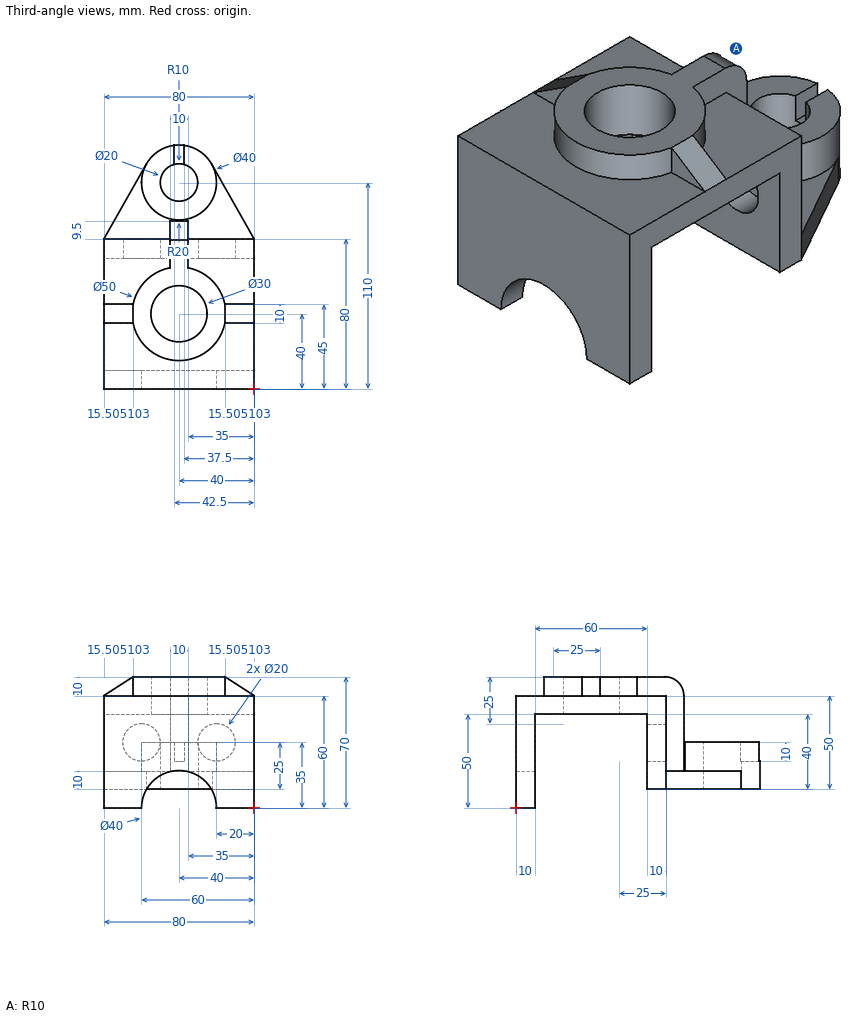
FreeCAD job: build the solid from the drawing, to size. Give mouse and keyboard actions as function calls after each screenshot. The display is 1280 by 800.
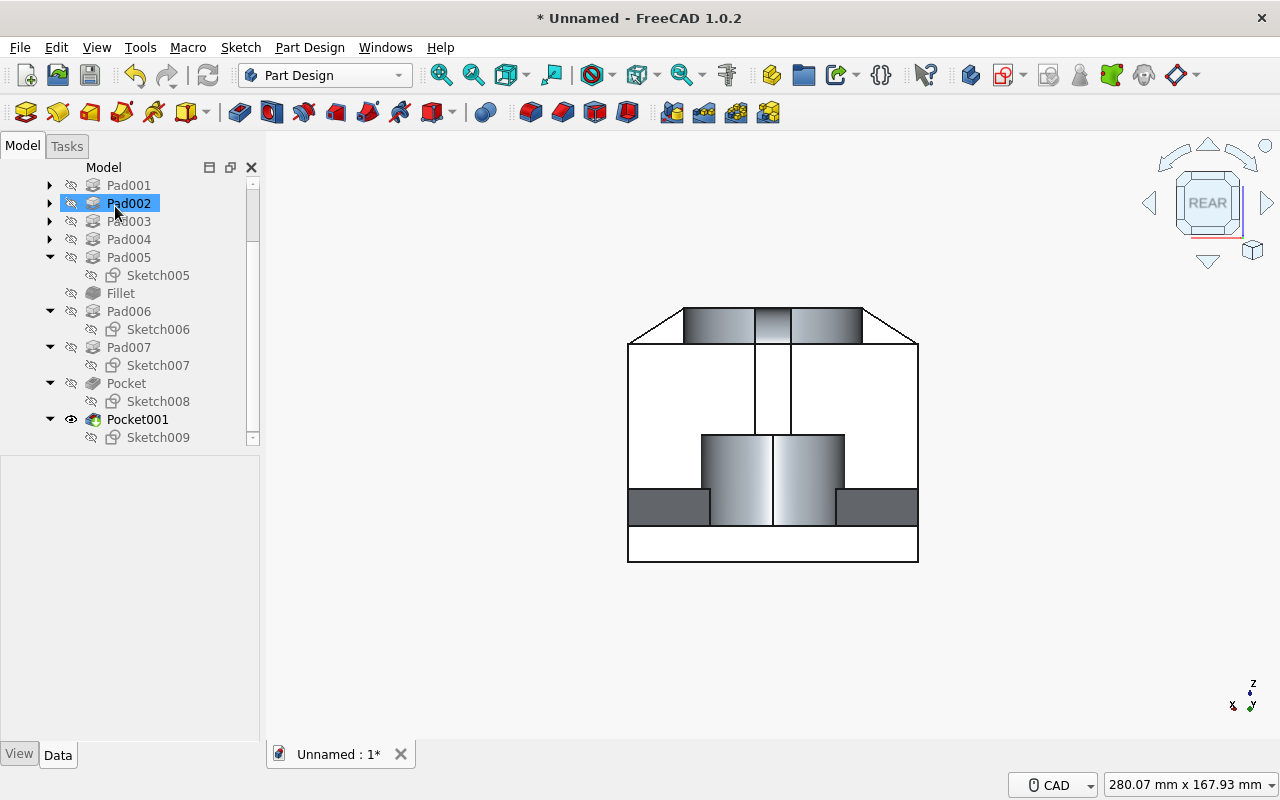
click(442, 76)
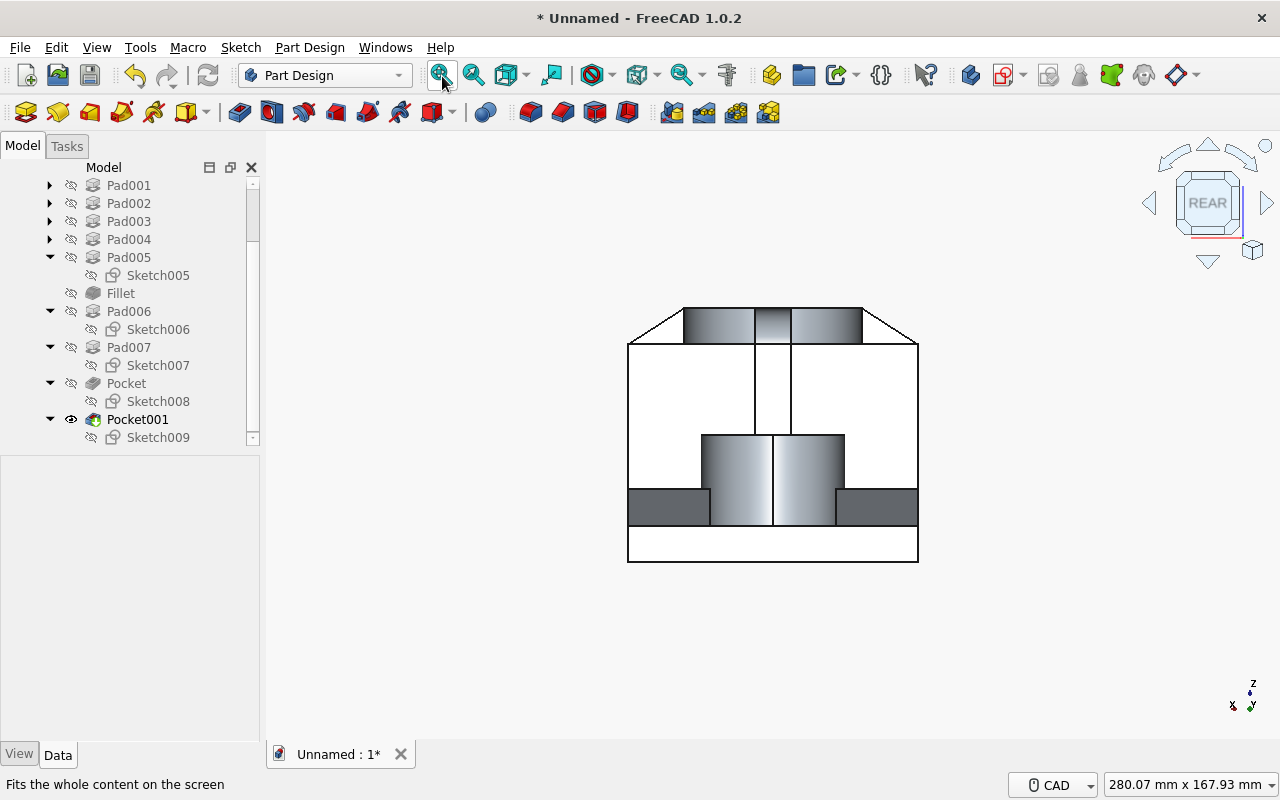
click(692, 416)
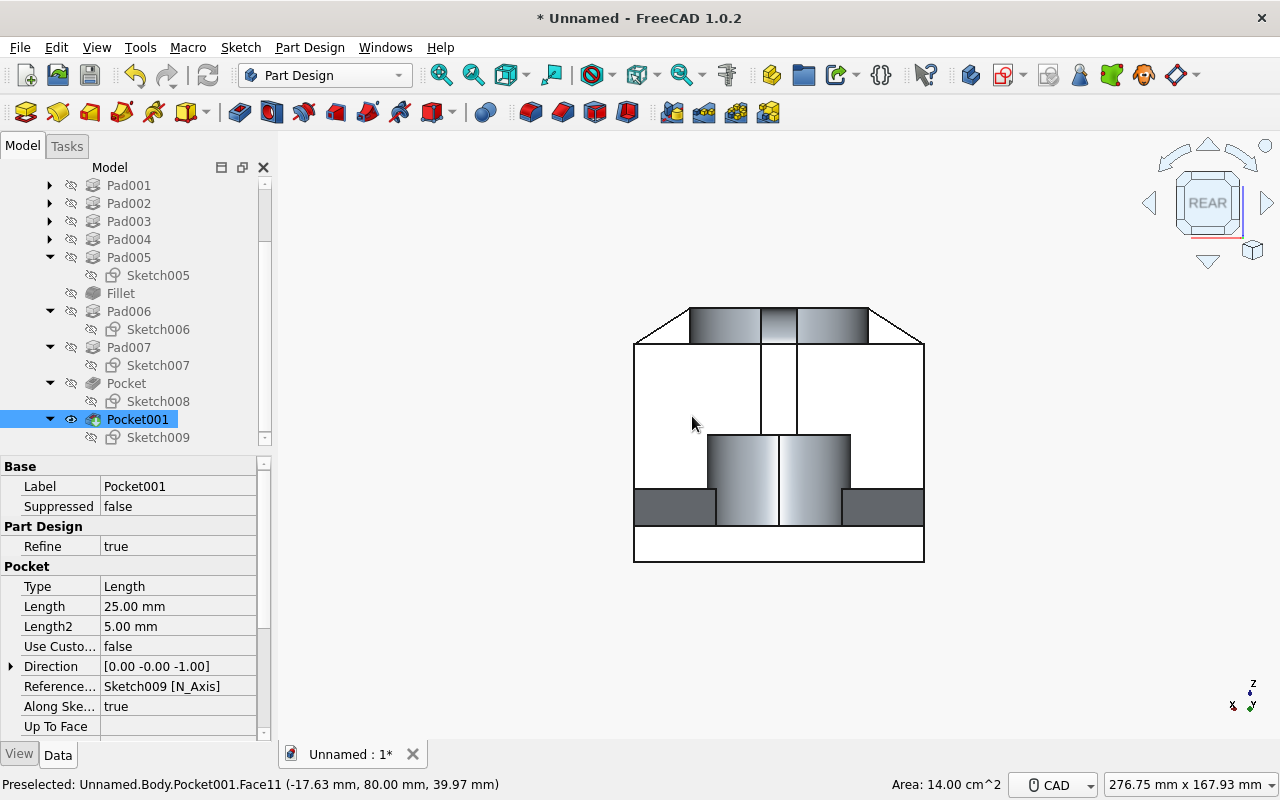
click(1004, 76)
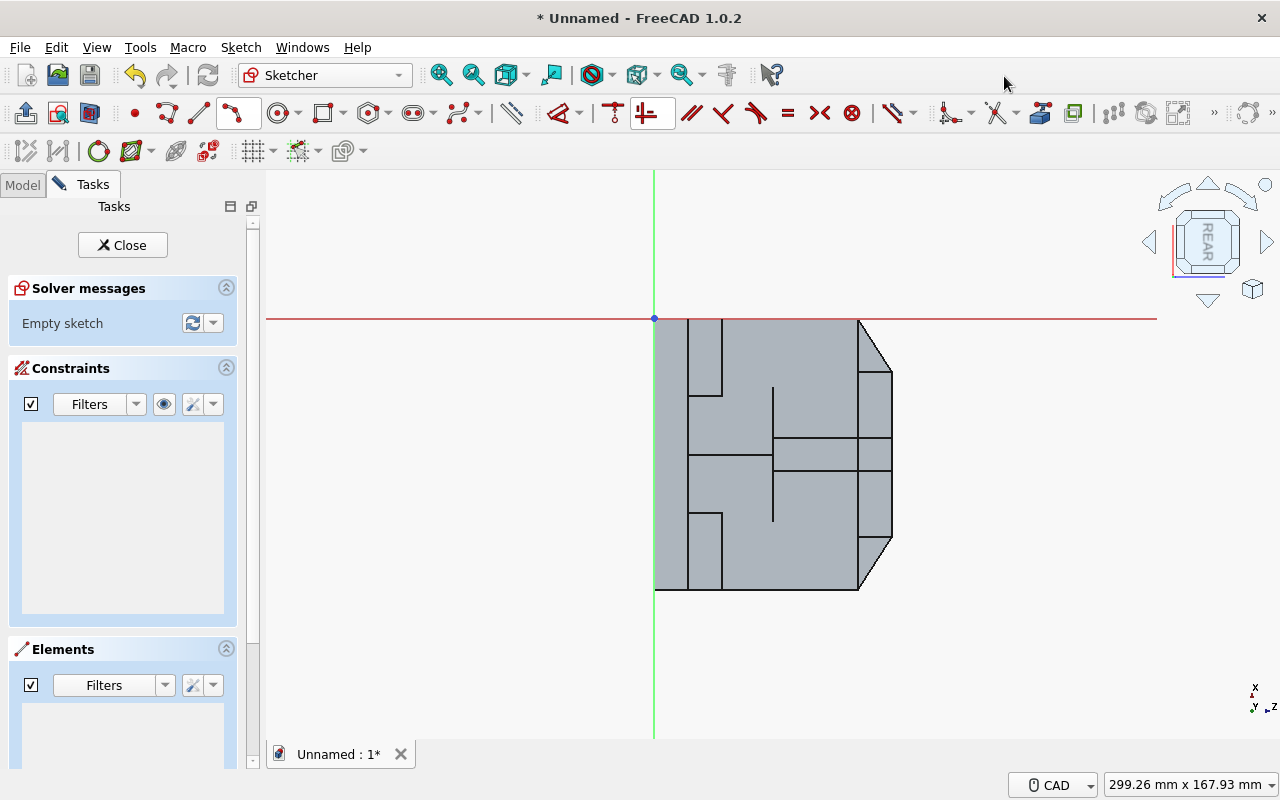
scroll(784, 403, up, 2)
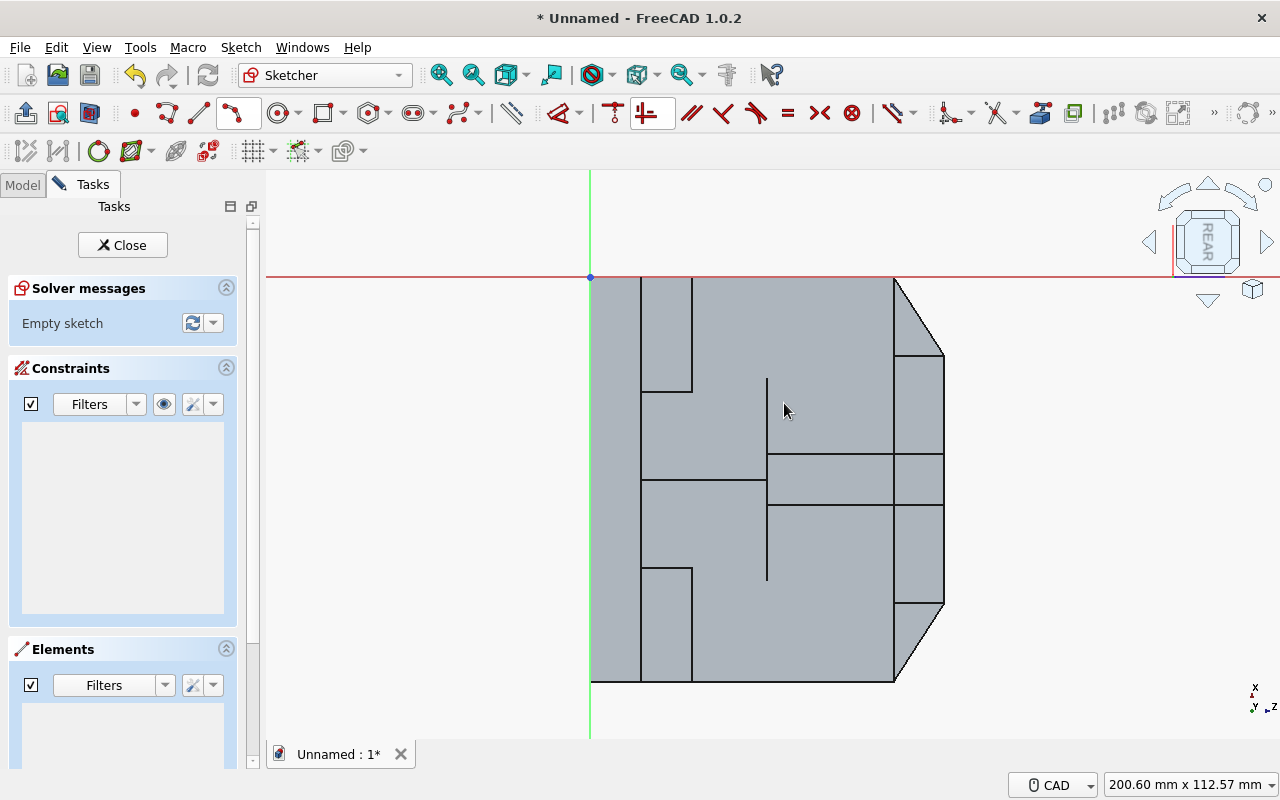
click(278, 114)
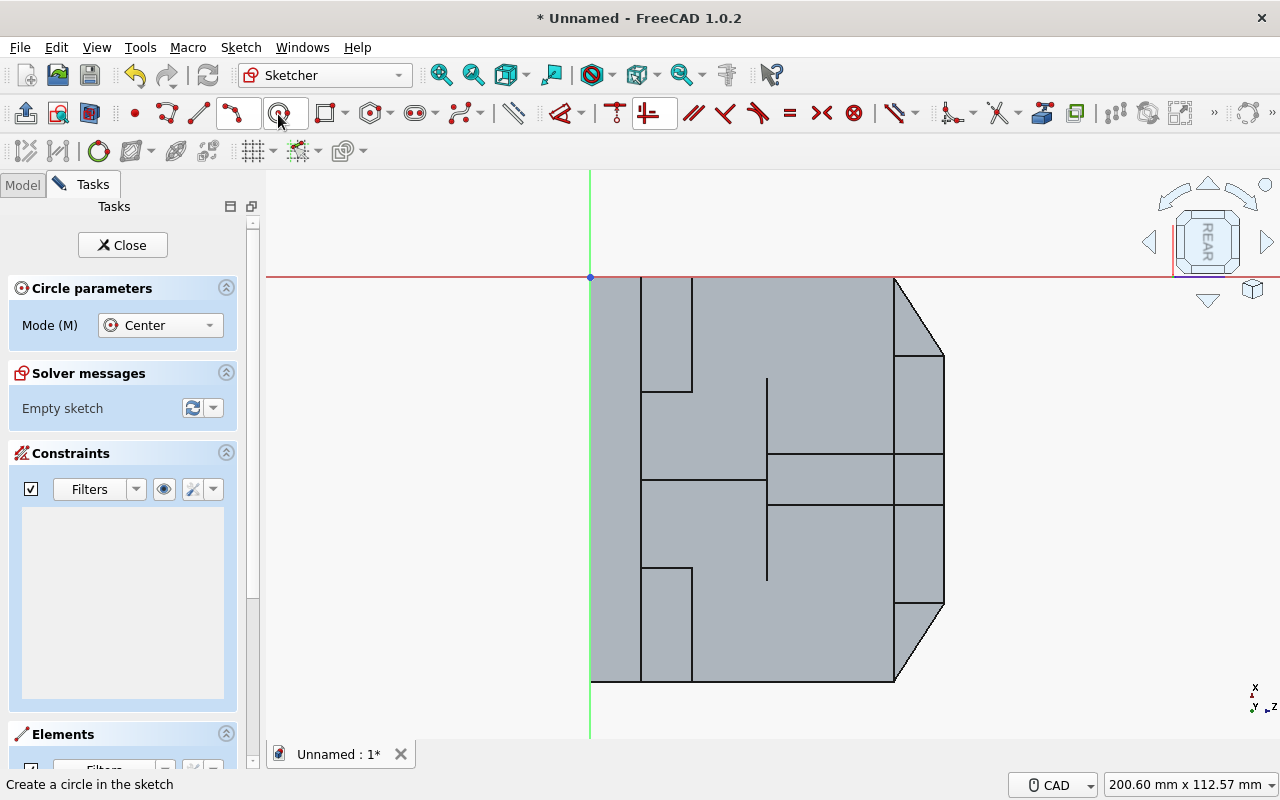
click(767, 379)
move(803, 343)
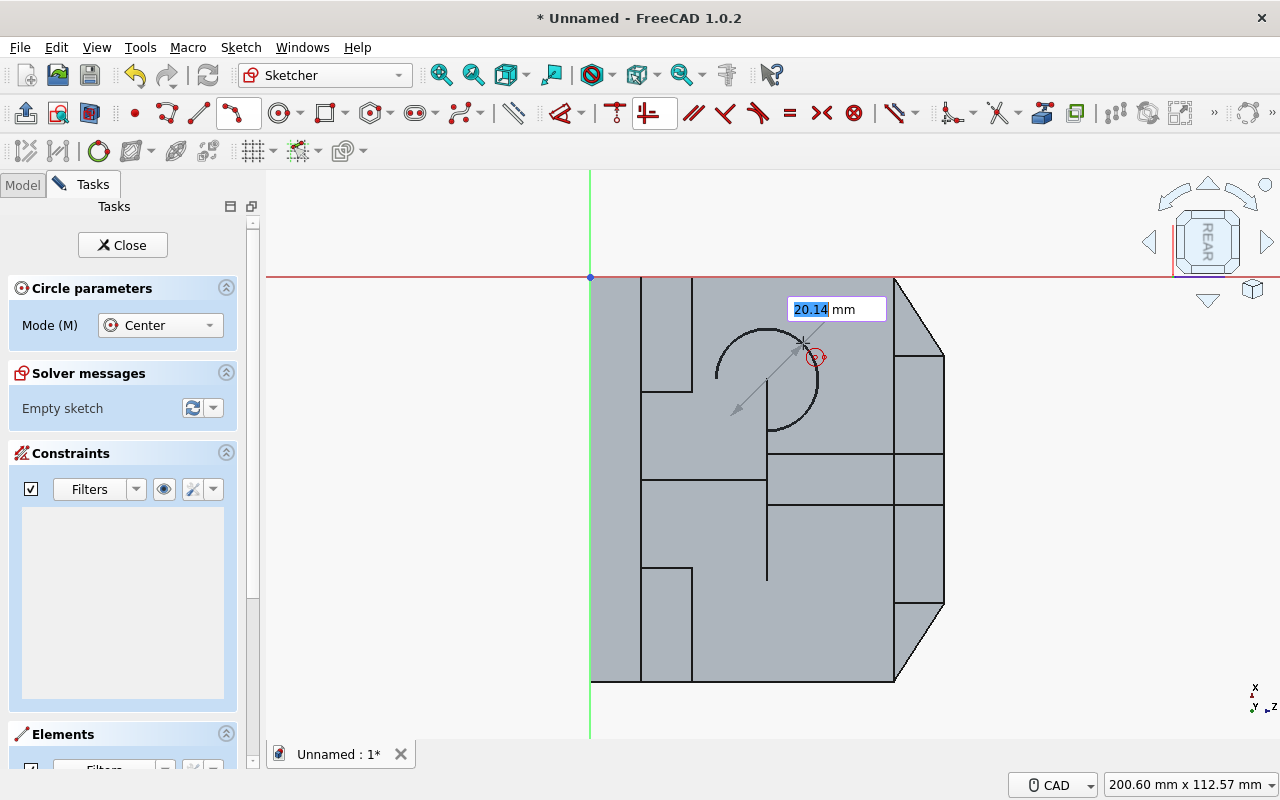
text(20)
key(Return)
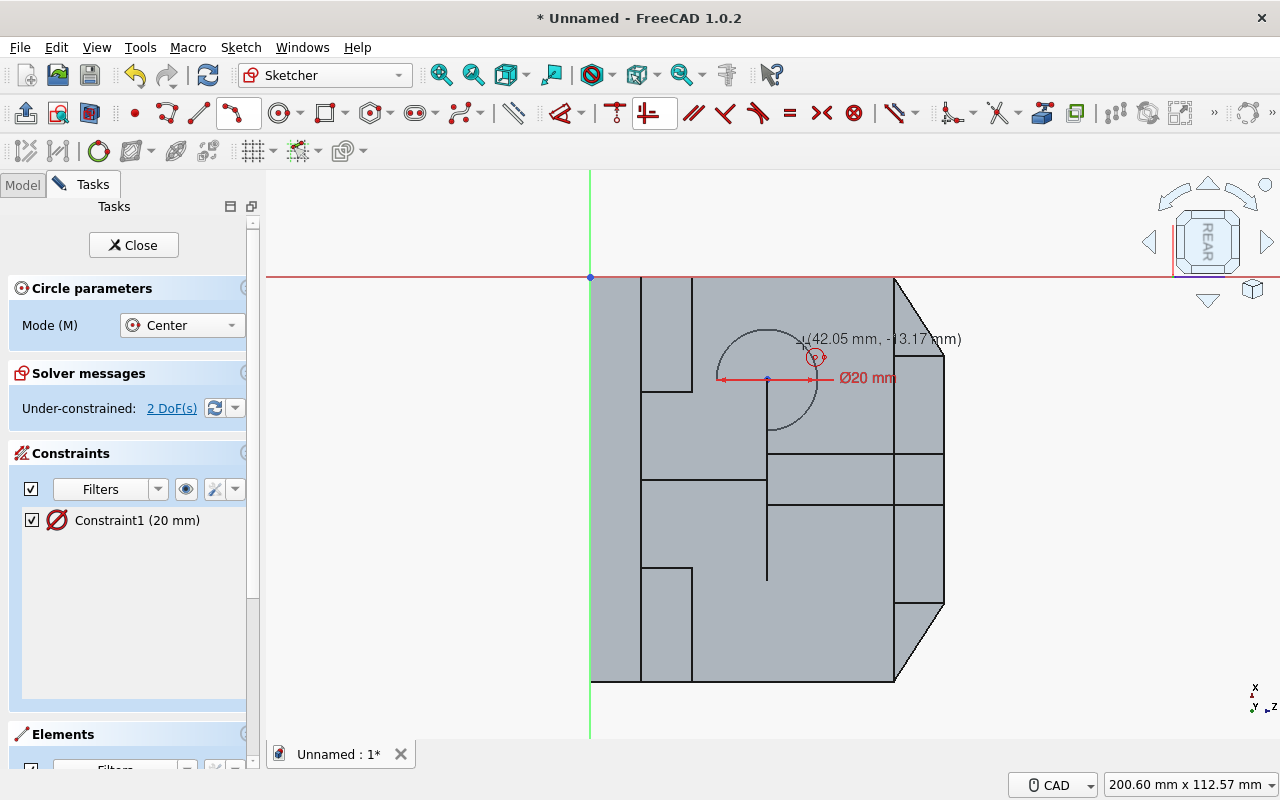
click(767, 581)
move(803, 545)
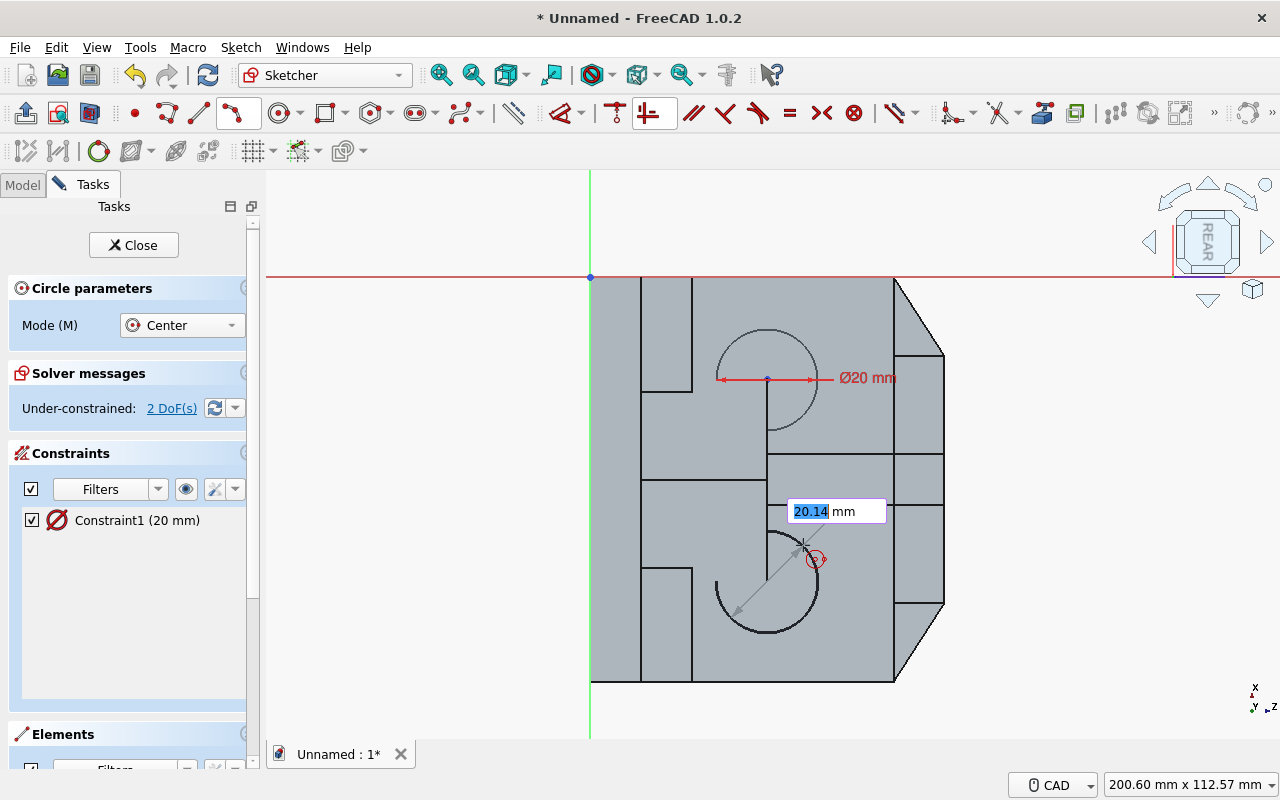
text(20)
key(Return)
key(Escape)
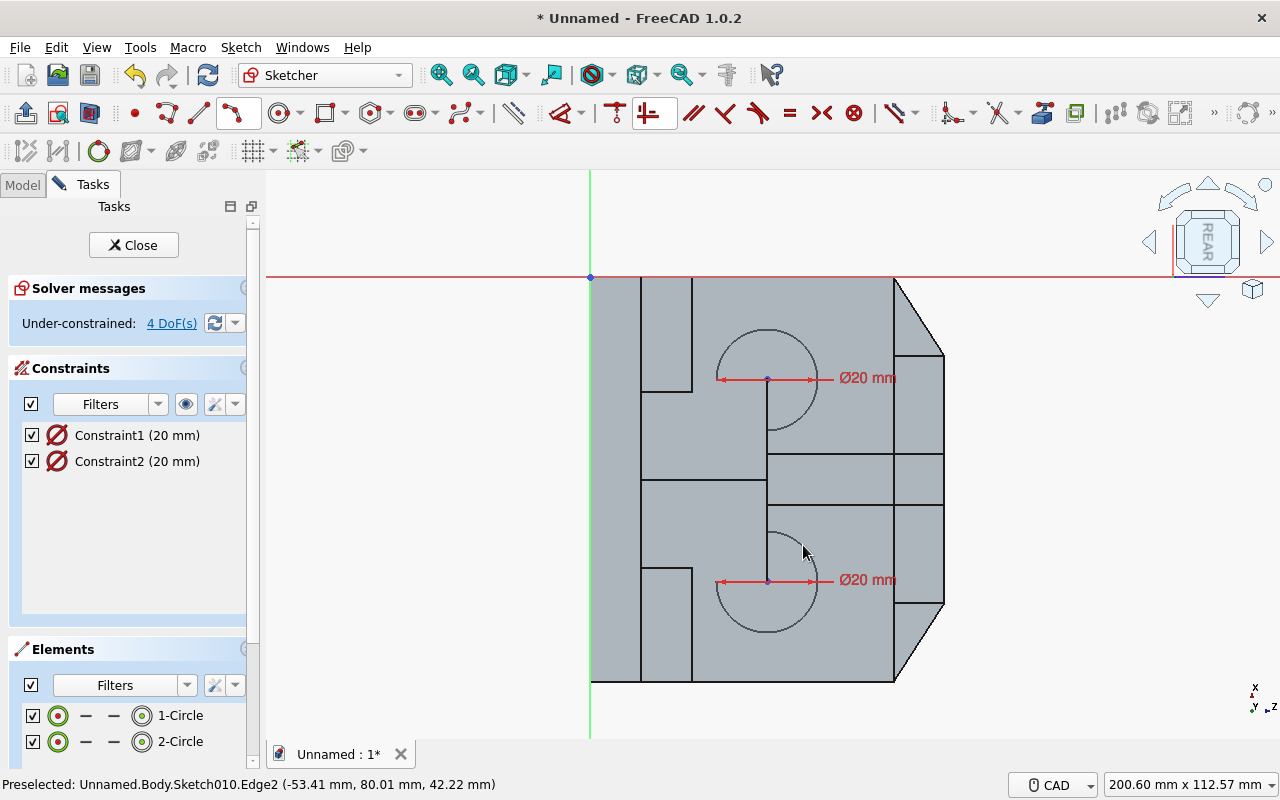
click(767, 380)